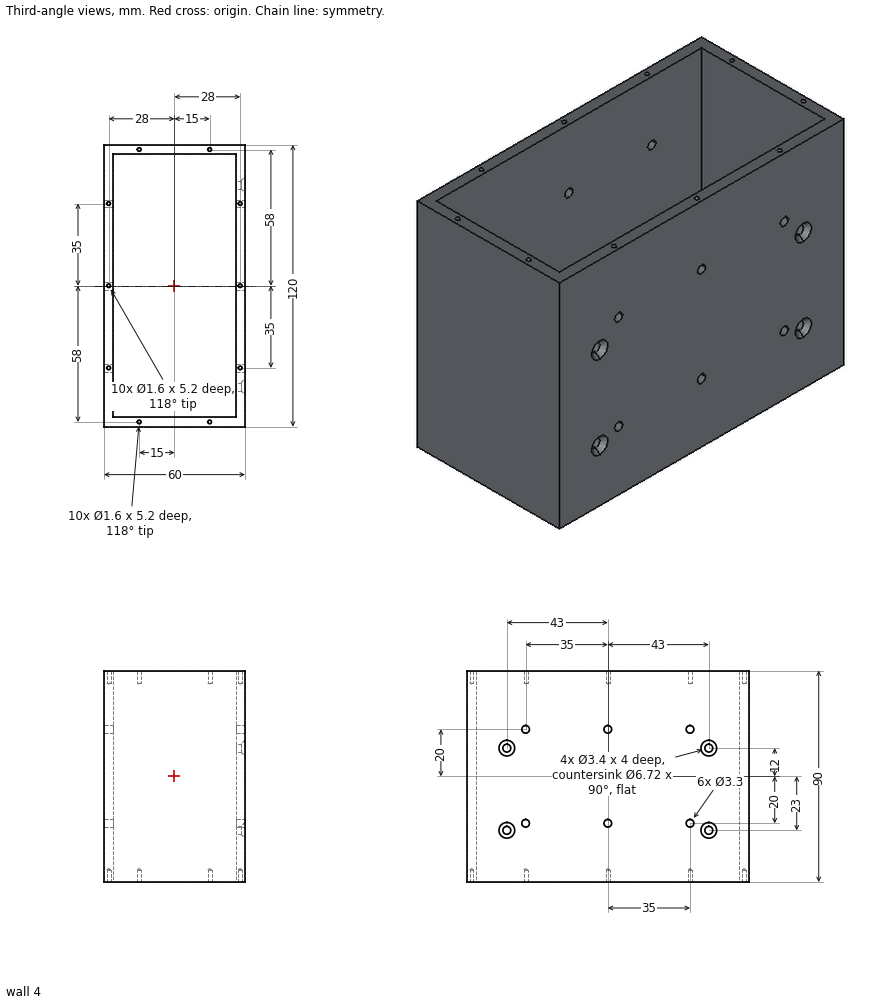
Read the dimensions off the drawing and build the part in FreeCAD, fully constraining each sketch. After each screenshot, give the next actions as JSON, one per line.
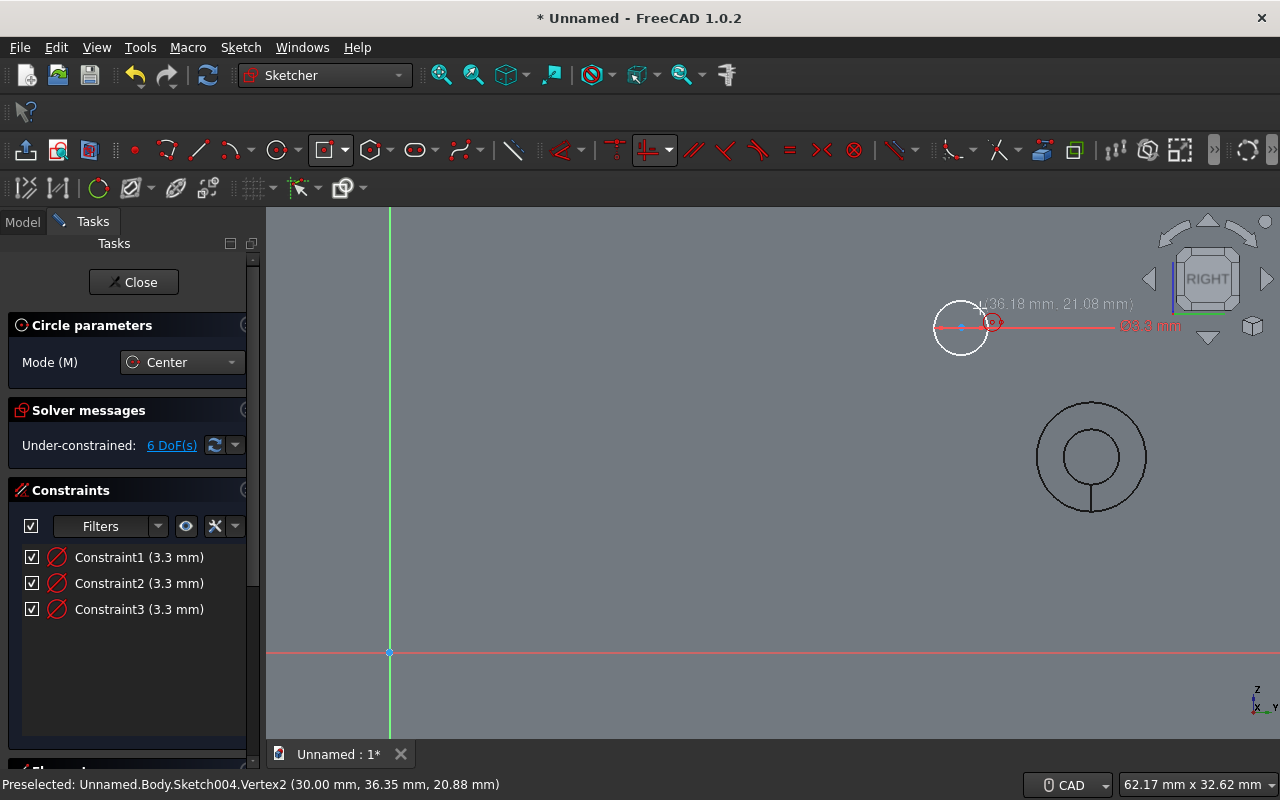
{"action": "scroll", "coordinate": [961, 326], "scroll_direction": "down", "scroll_amount": 4}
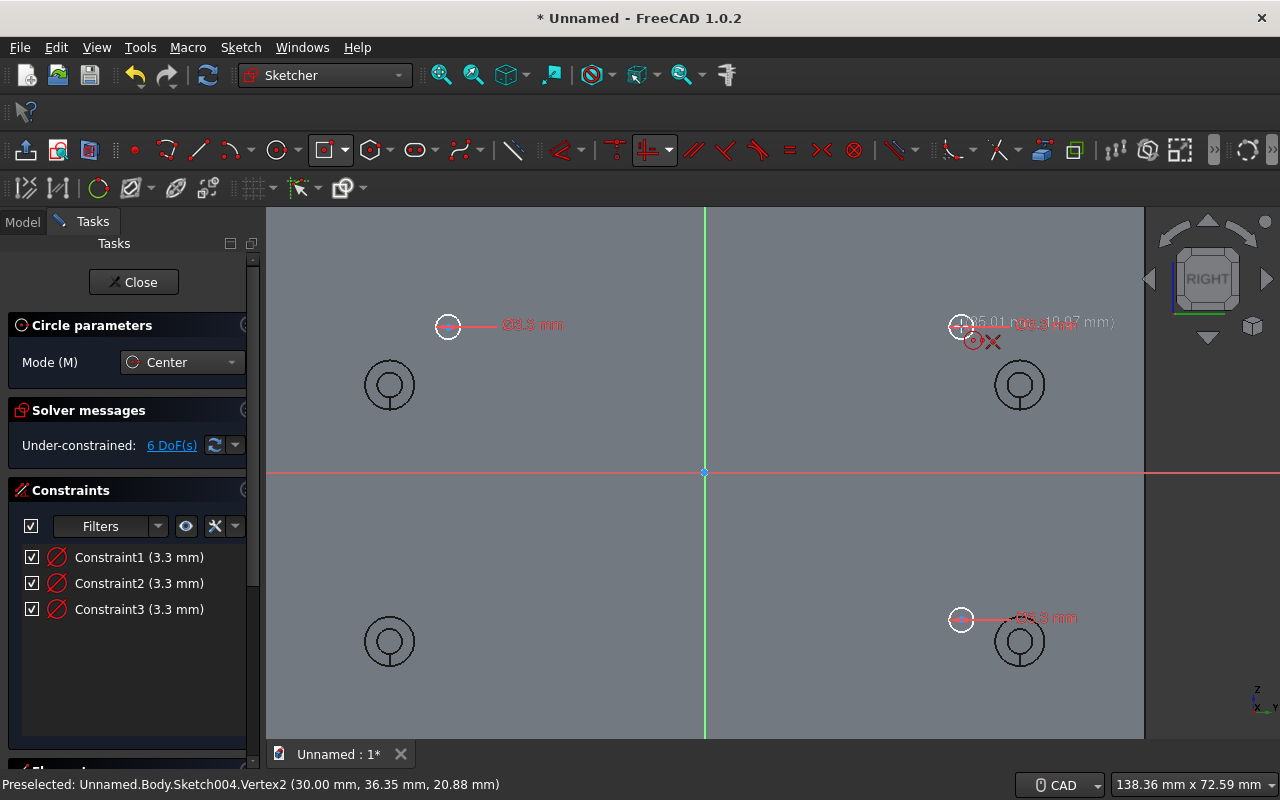
{"action": "scroll", "coordinate": [448, 620], "scroll_direction": "up", "scroll_amount": 4}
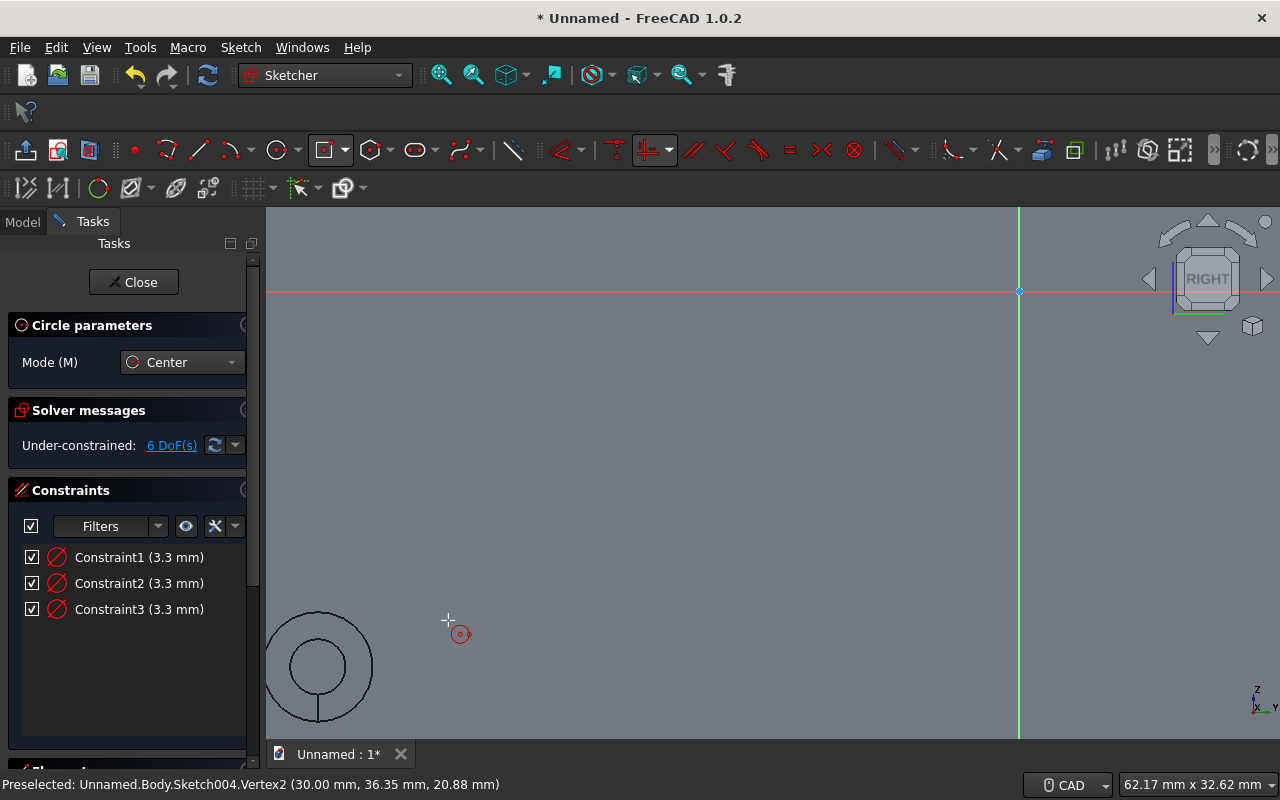
{"action": "left_click", "coordinate": [448, 618]}
{"action": "mouse_move", "coordinate": [467, 599]}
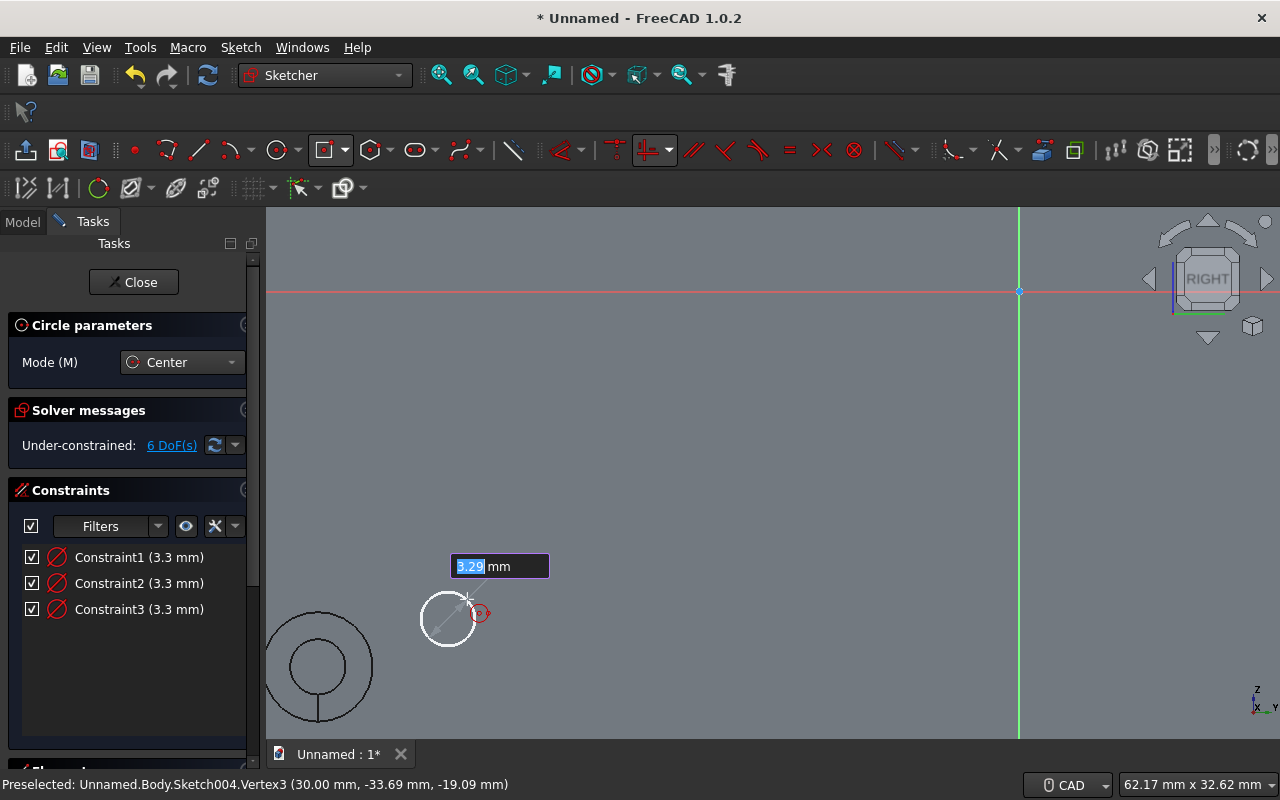
{"action": "type", "text": "3.3"}
{"action": "key", "text": "Return"}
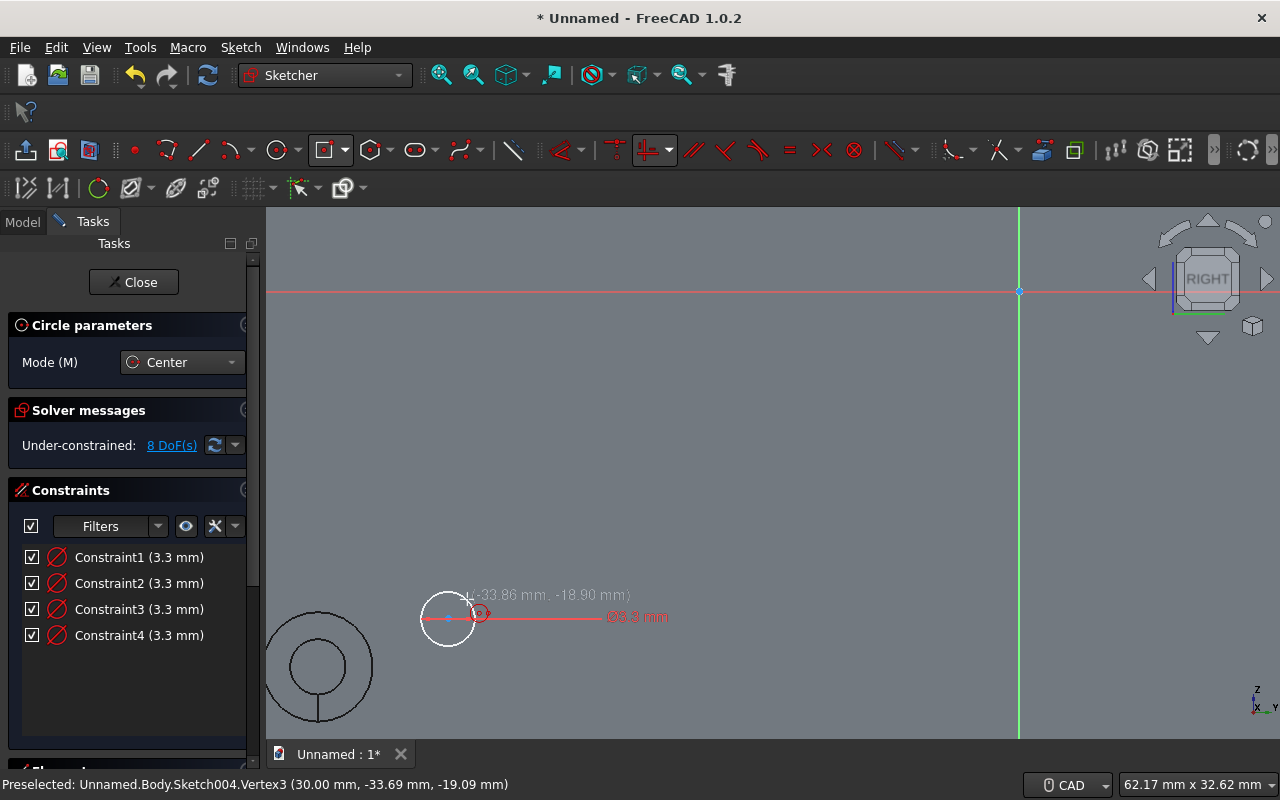
{"action": "scroll", "coordinate": [448, 621], "scroll_direction": "down", "scroll_amount": 4}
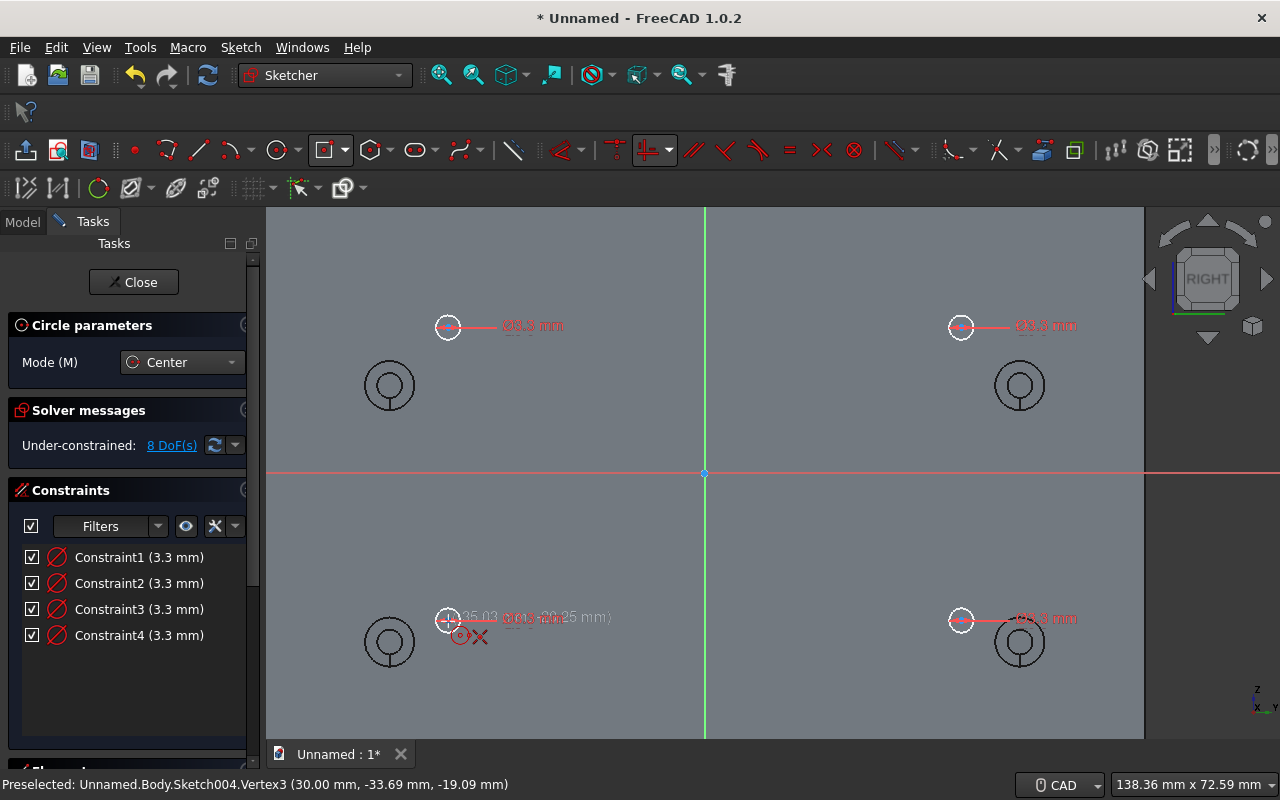
{"action": "scroll", "coordinate": [705, 327], "scroll_direction": "up", "scroll_amount": 4}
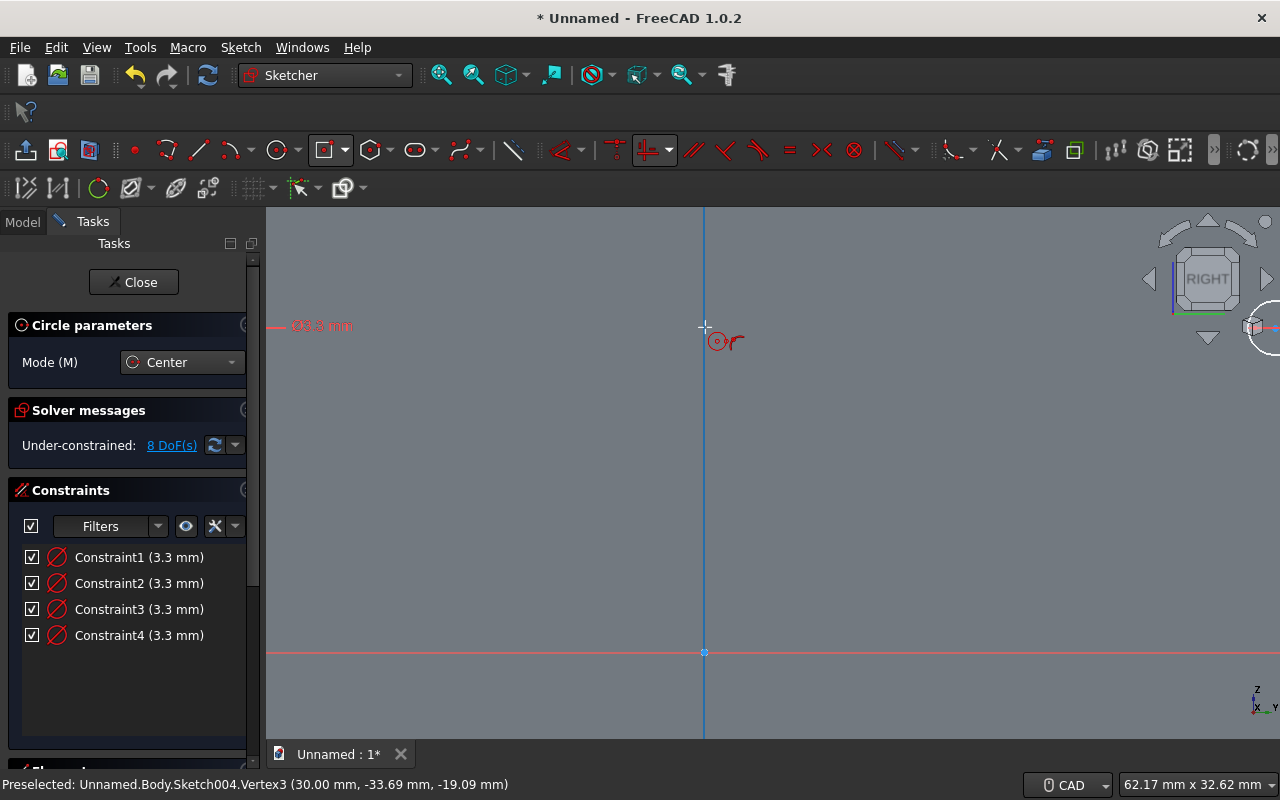
{"action": "left_click", "coordinate": [704, 327]}
{"action": "mouse_move", "coordinate": [723, 308]}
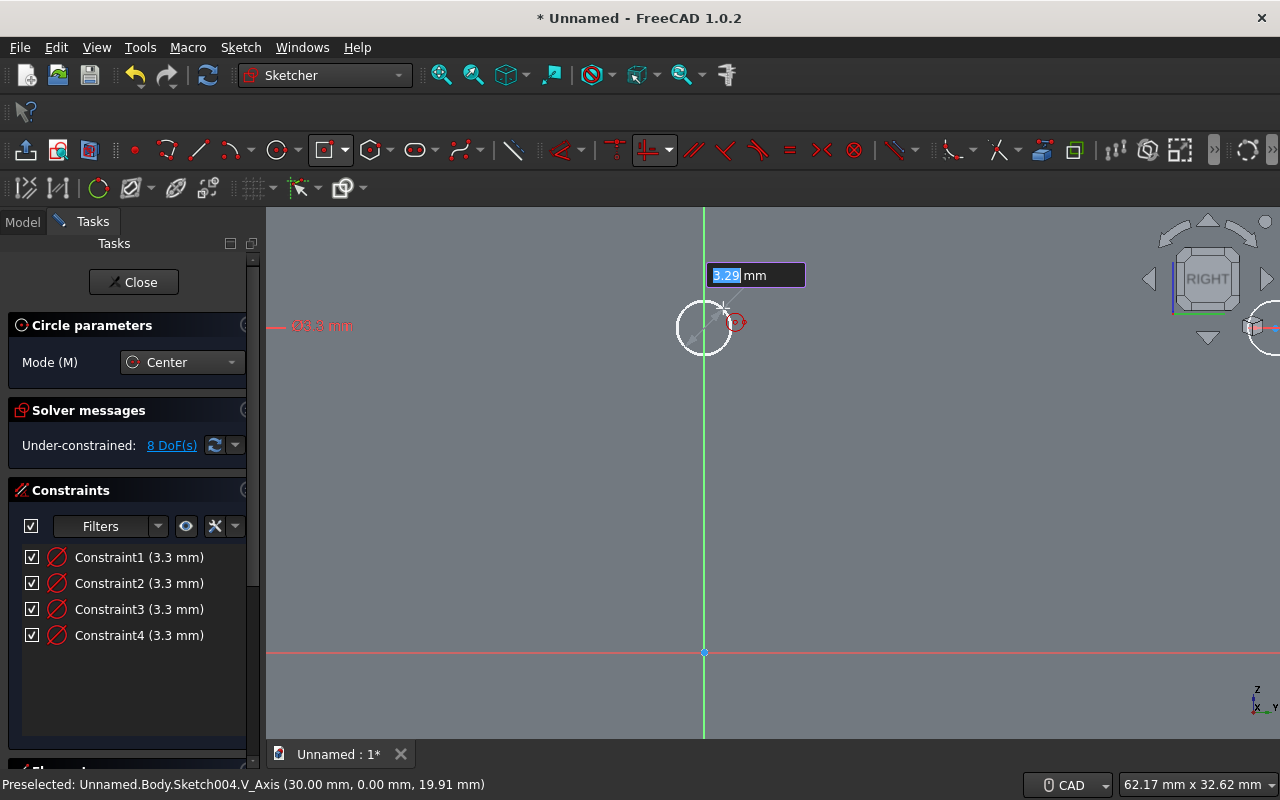
{"action": "type", "text": "3.3"}
{"action": "key", "text": "Return"}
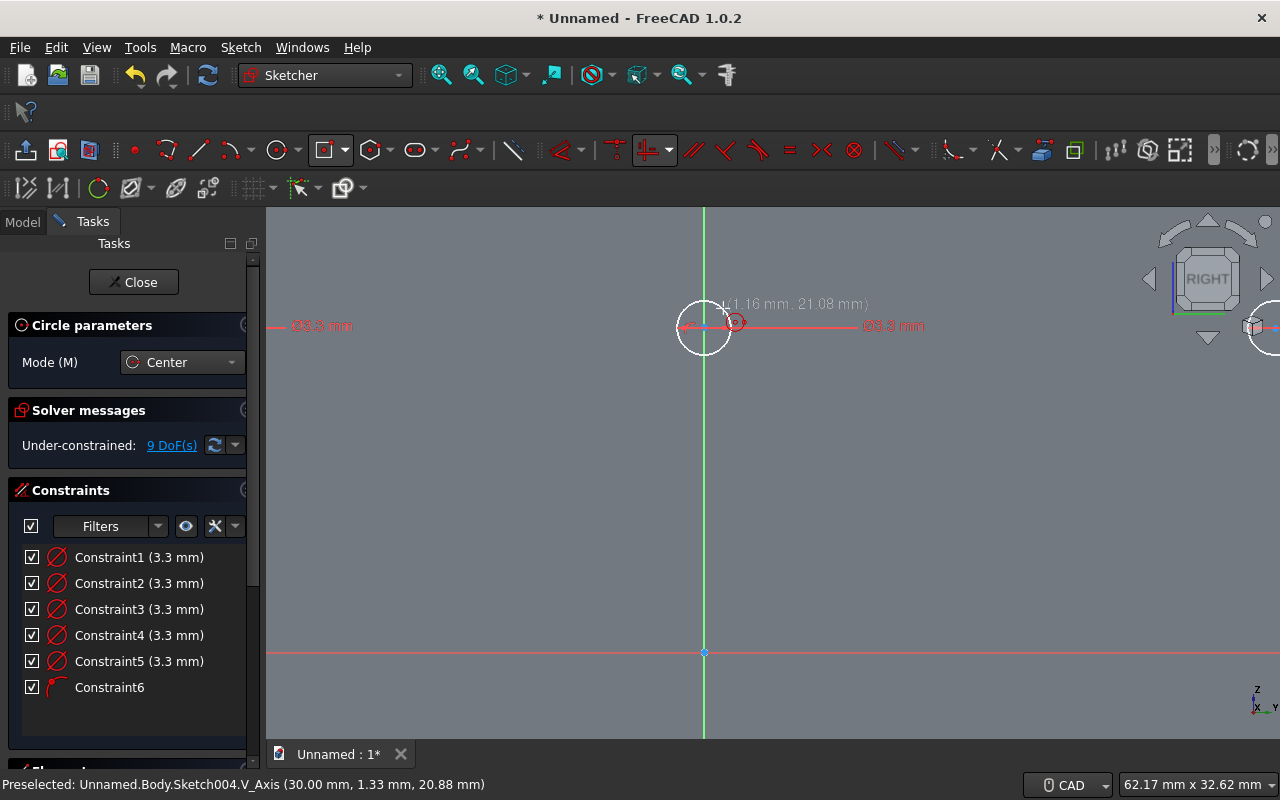
{"action": "scroll", "coordinate": [705, 326], "scroll_direction": "down", "scroll_amount": 4}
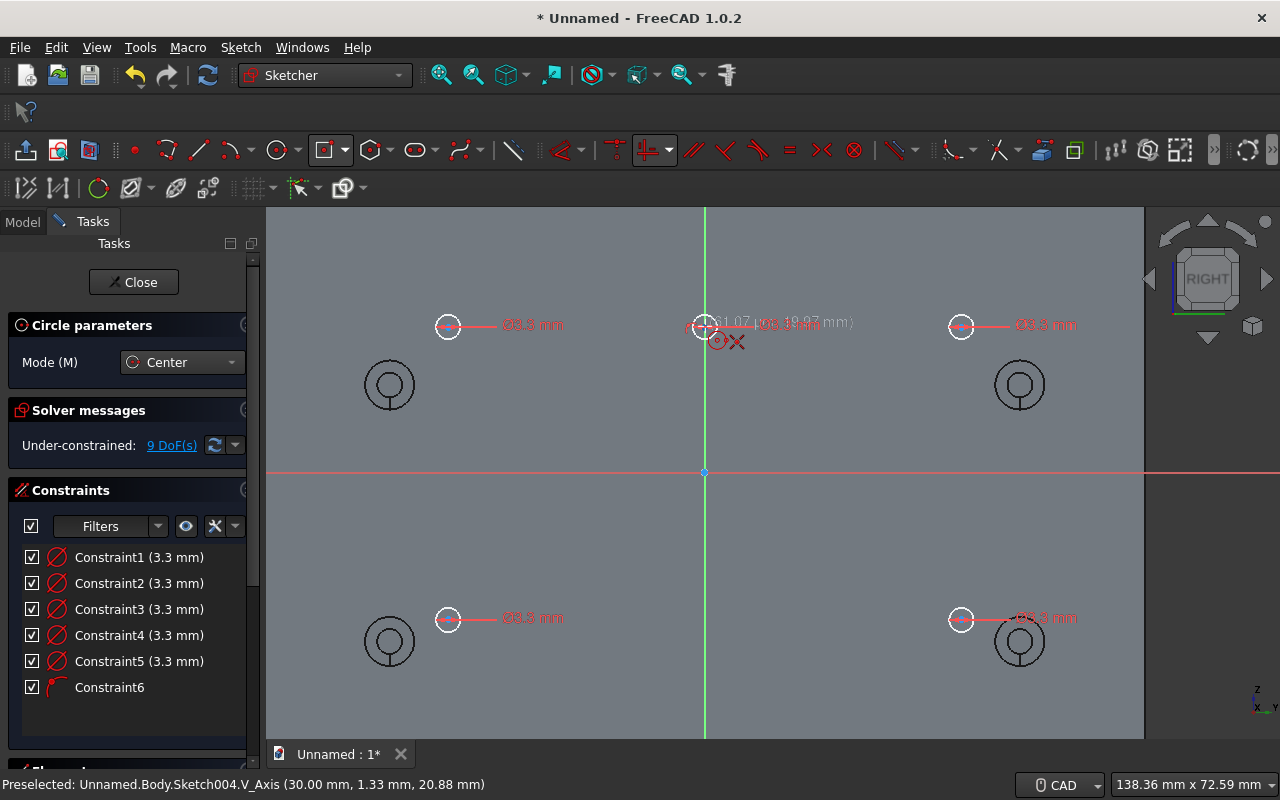
{"action": "scroll", "coordinate": [705, 620], "scroll_direction": "up", "scroll_amount": 4}